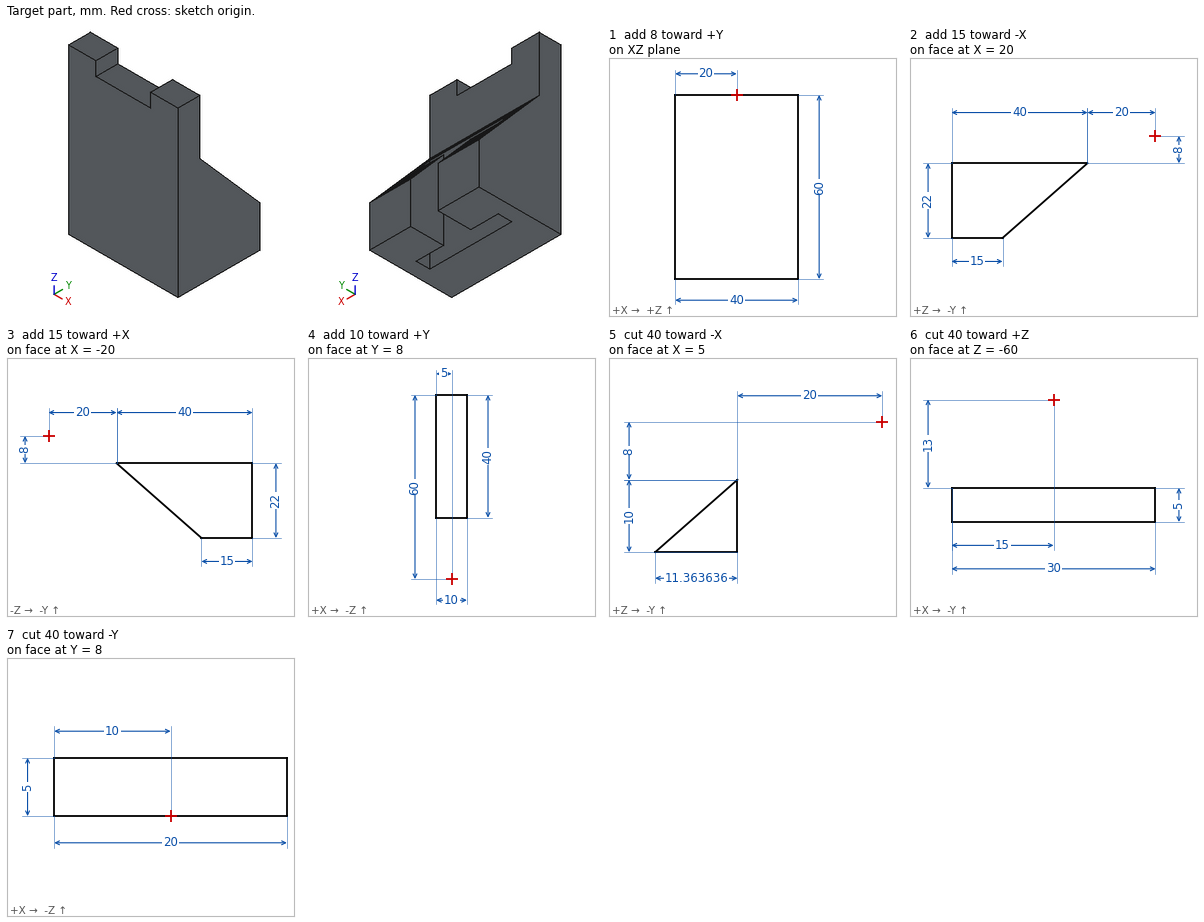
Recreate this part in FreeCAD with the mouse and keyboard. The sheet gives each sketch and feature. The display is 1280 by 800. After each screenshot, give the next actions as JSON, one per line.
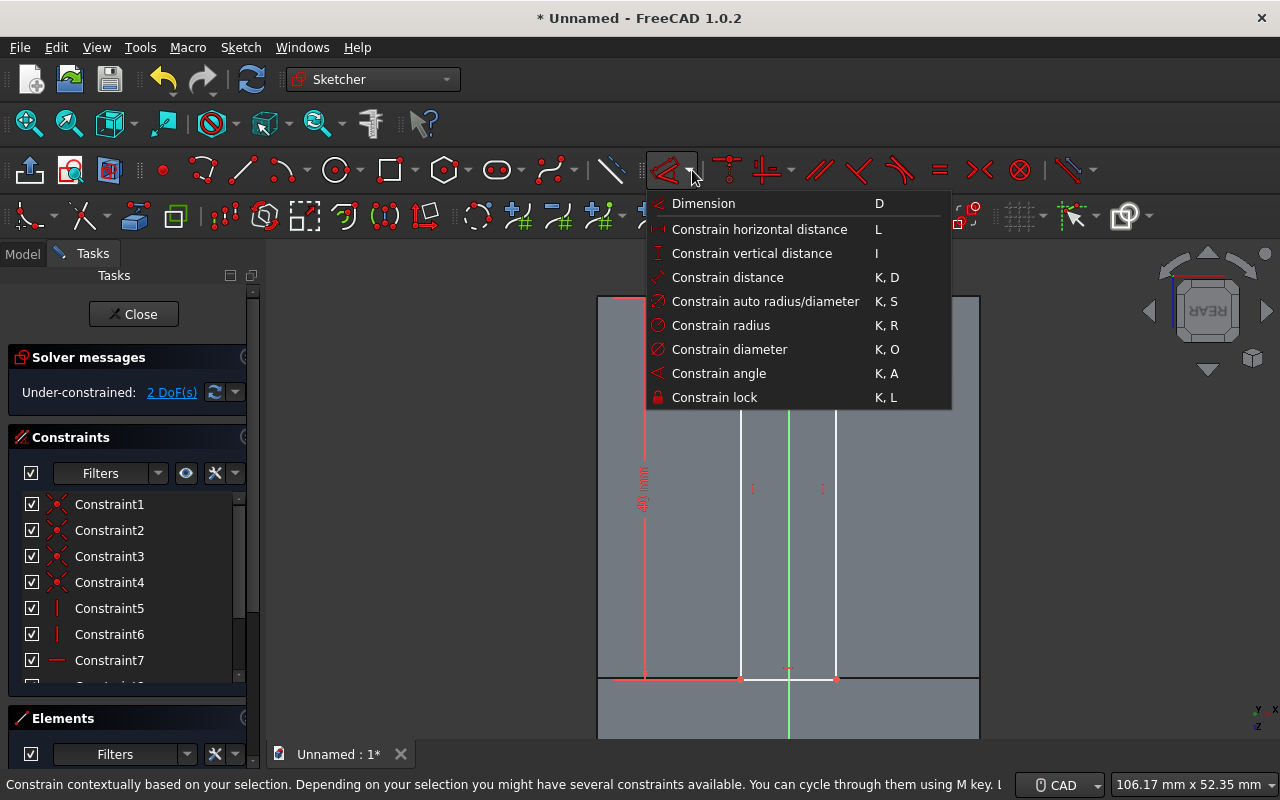
{"action": "left_click", "coordinate": [799, 229]}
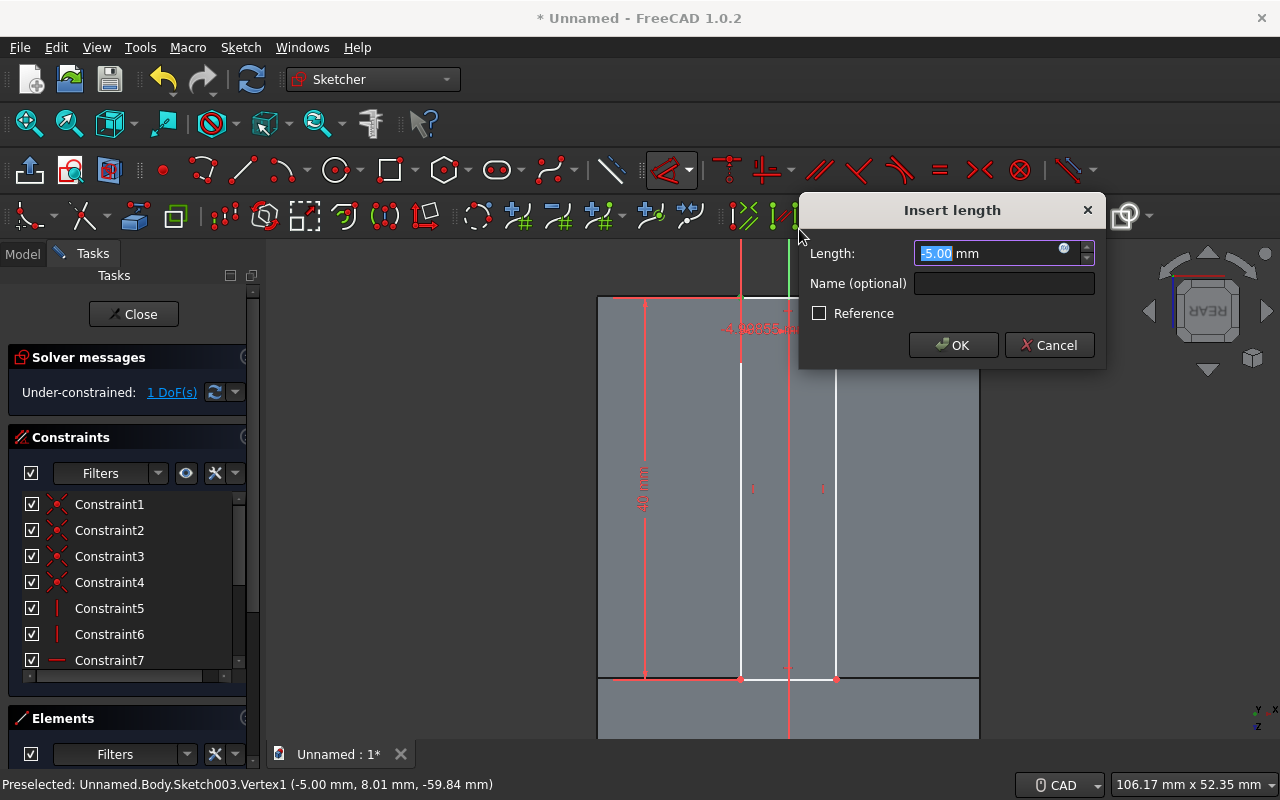
{"action": "type", "text": "-5"}
{"action": "key", "text": "Return"}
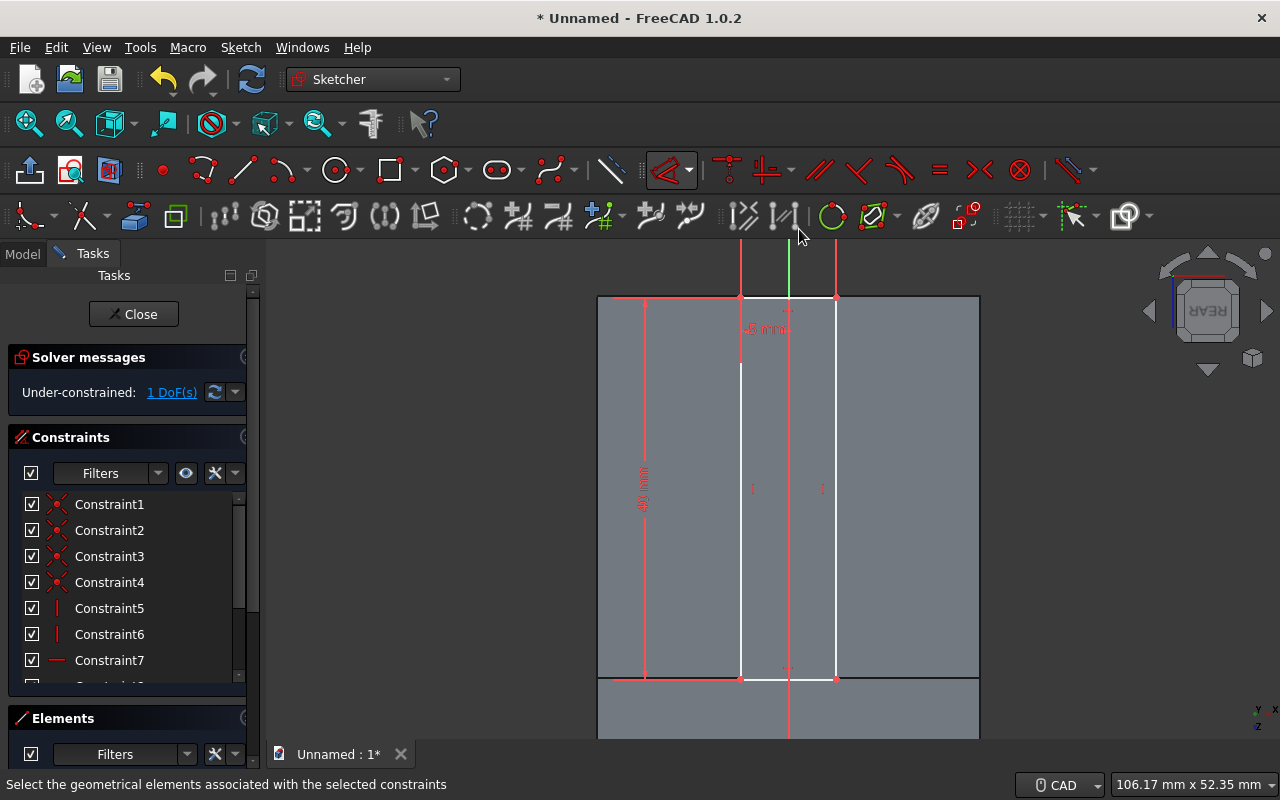
{"action": "left_click", "coordinate": [741, 298]}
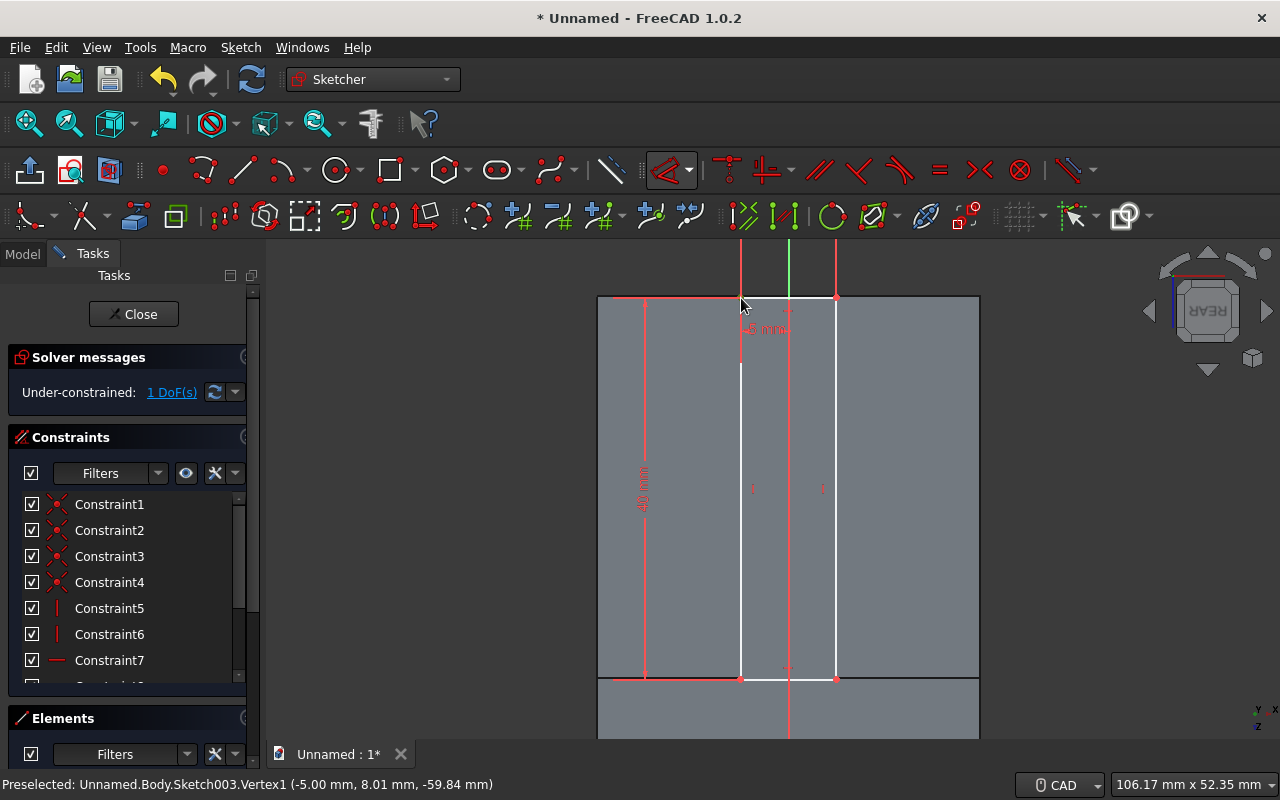
{"action": "key", "text": "i"}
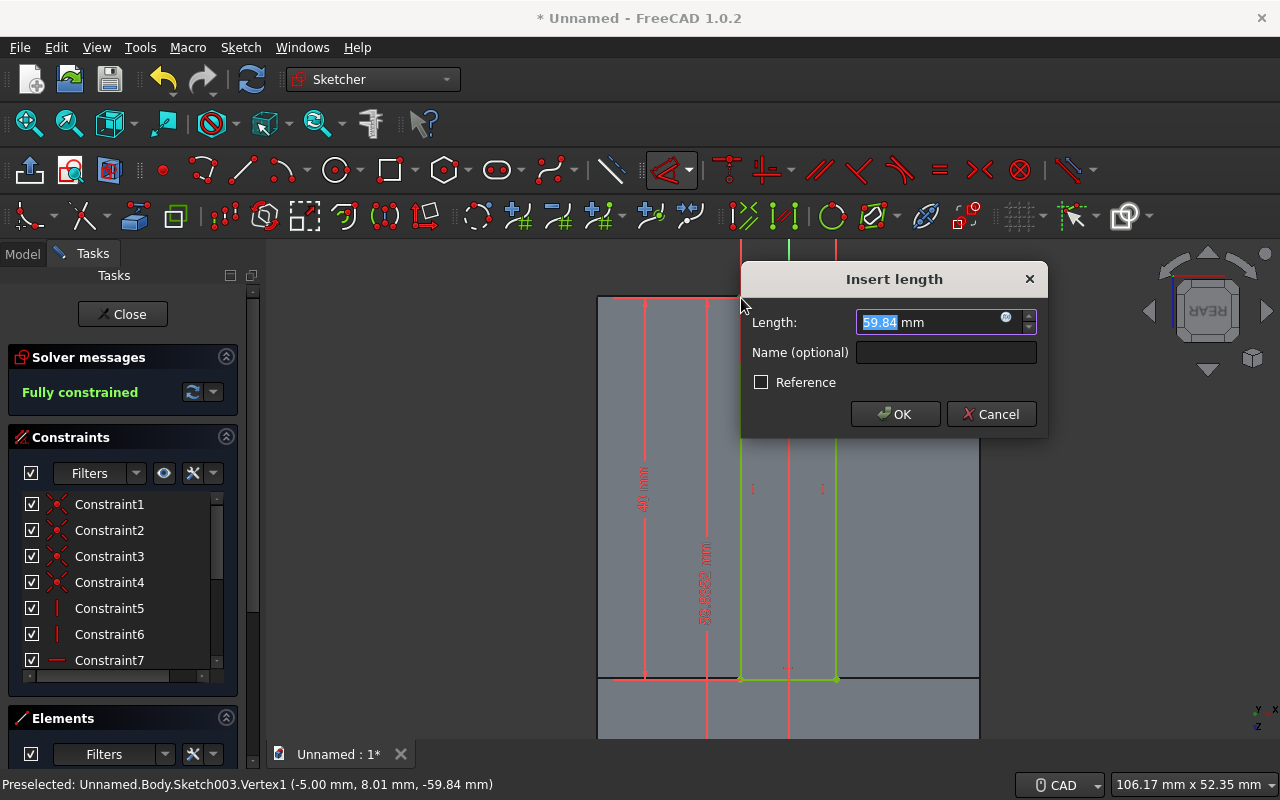
{"action": "type", "text": "60"}
{"action": "key", "text": "Return"}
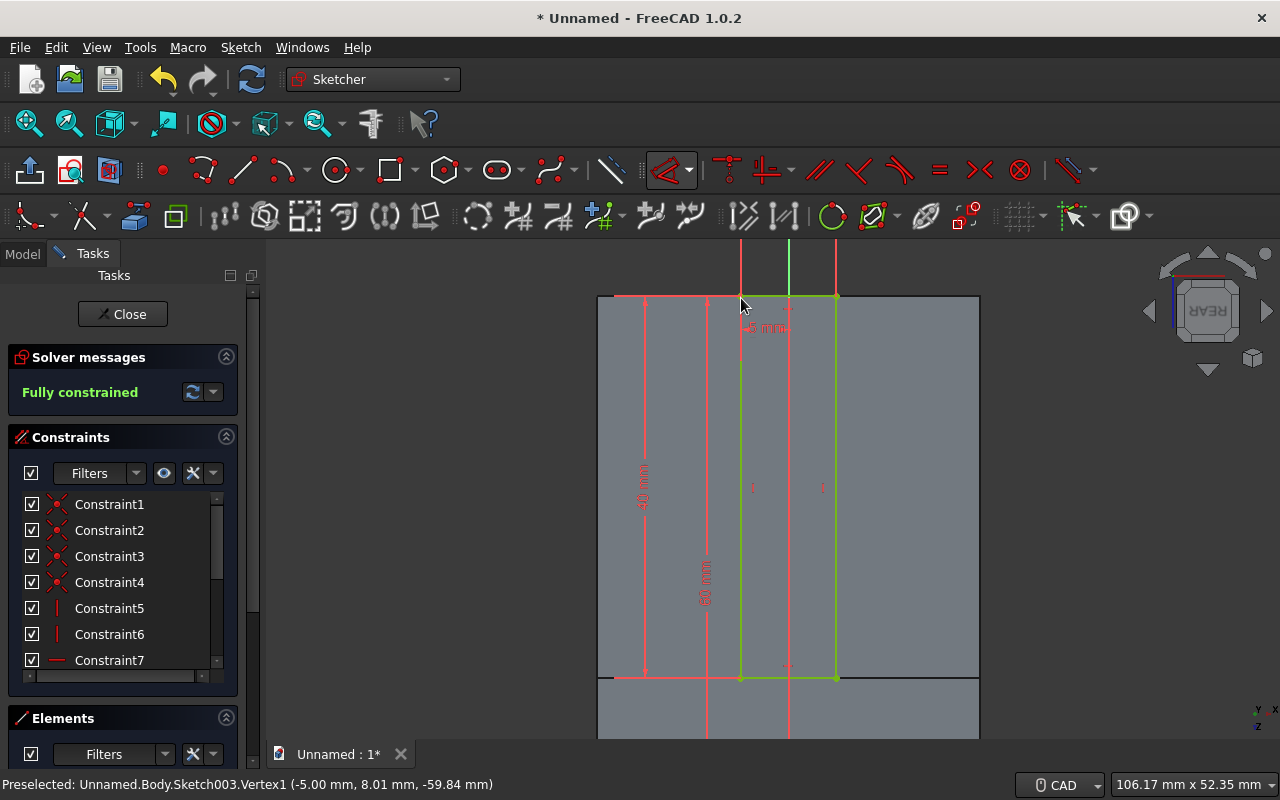
{"action": "left_click", "coordinate": [123, 314]}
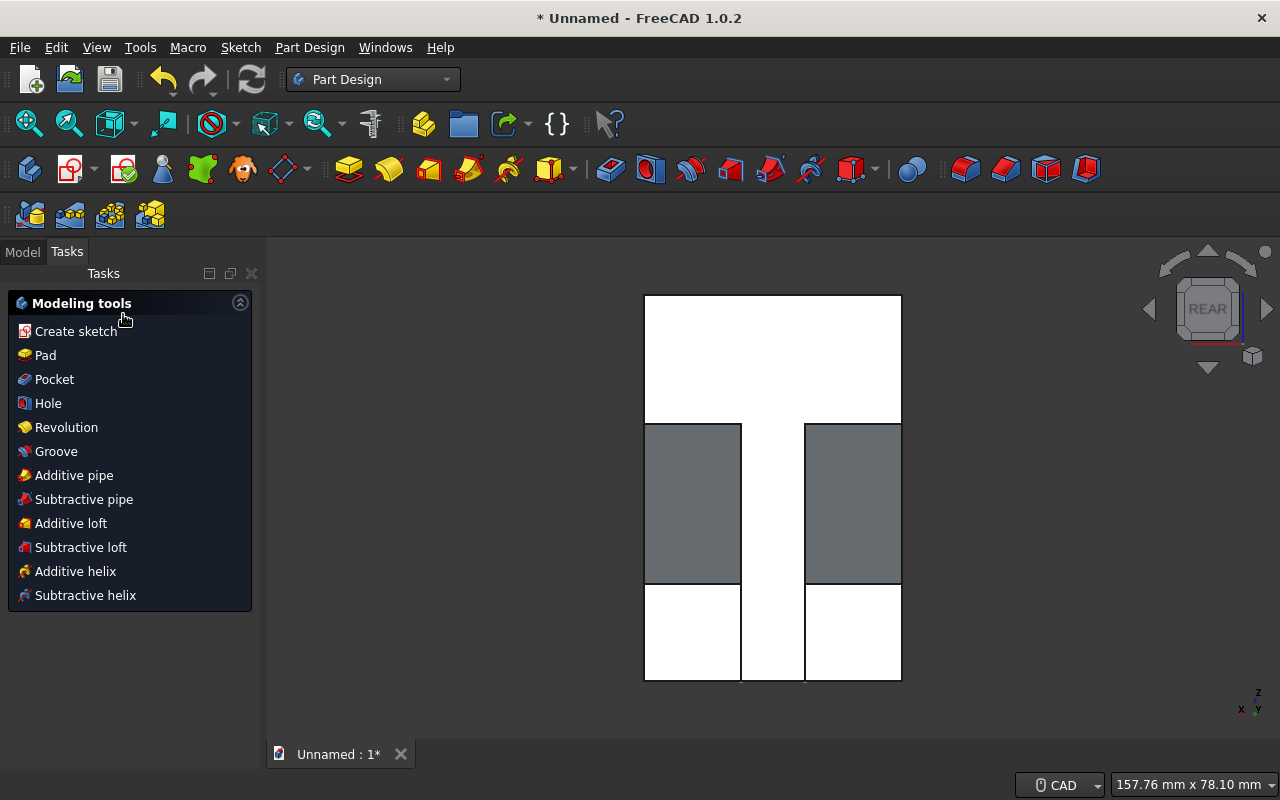
{"action": "left_click", "coordinate": [350, 170]}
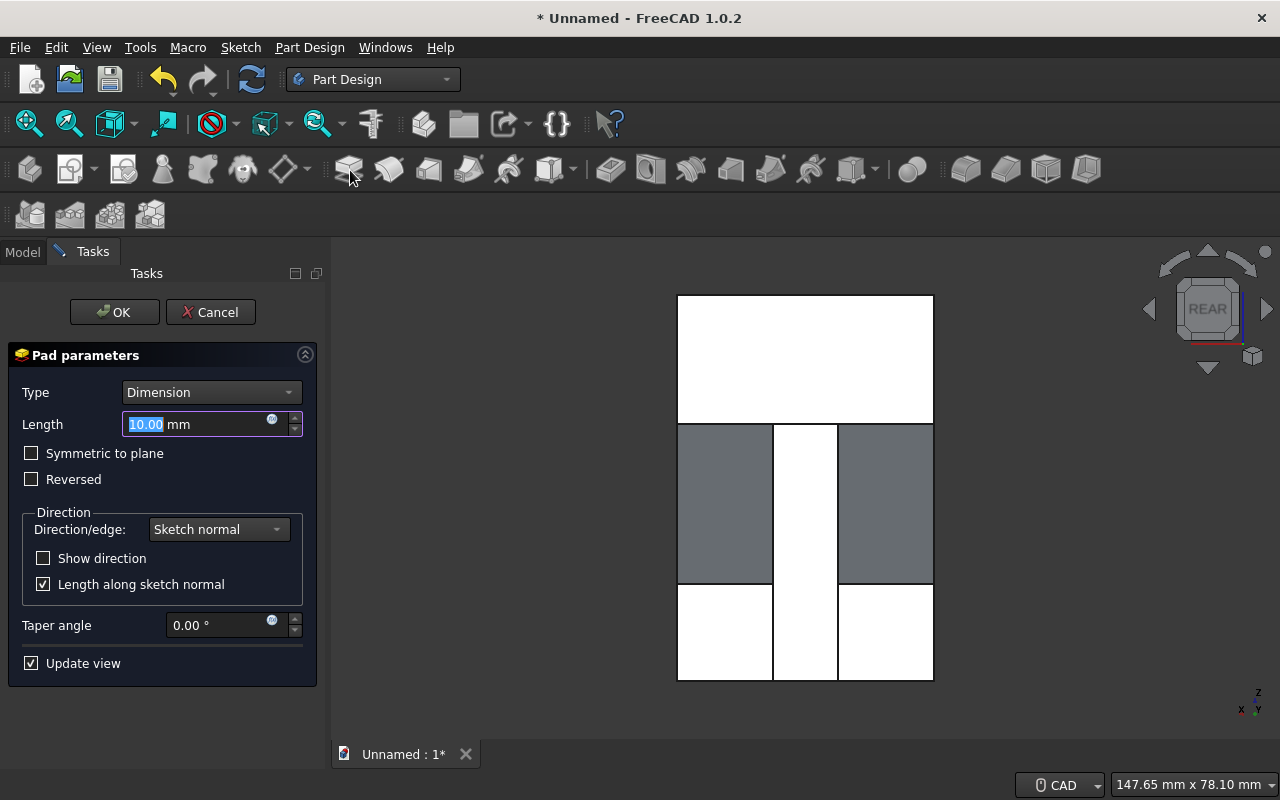
{"action": "type", "text": "10"}
{"action": "key", "text": "Tab"}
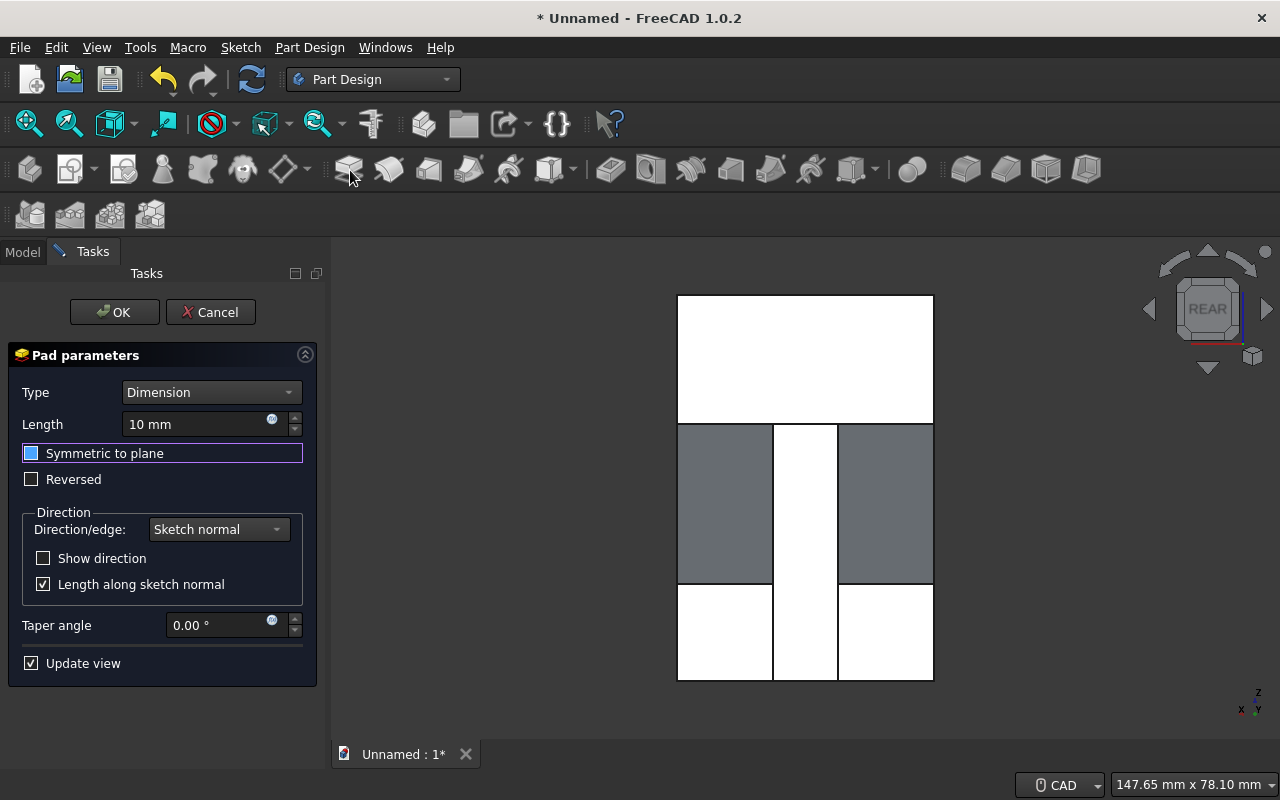
{"action": "left_click", "coordinate": [115, 312]}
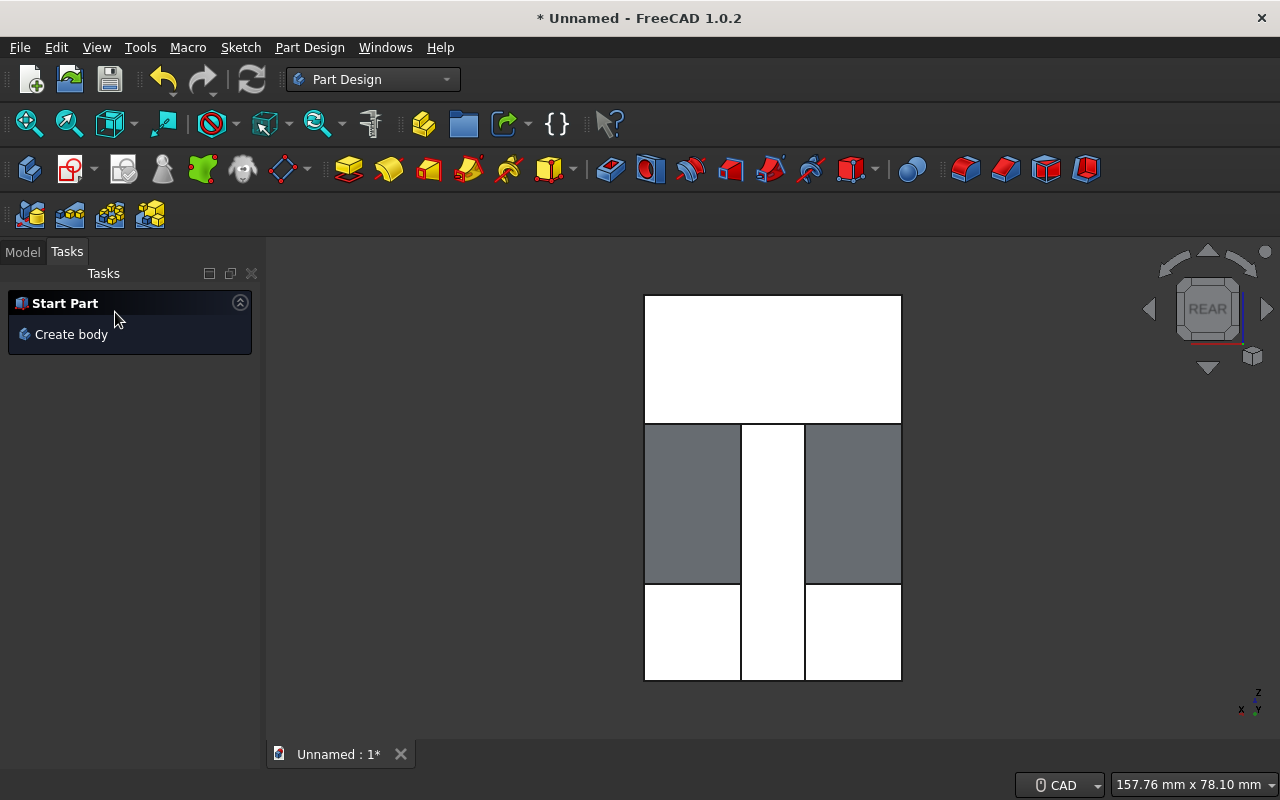
{"action": "key", "text": "0"}